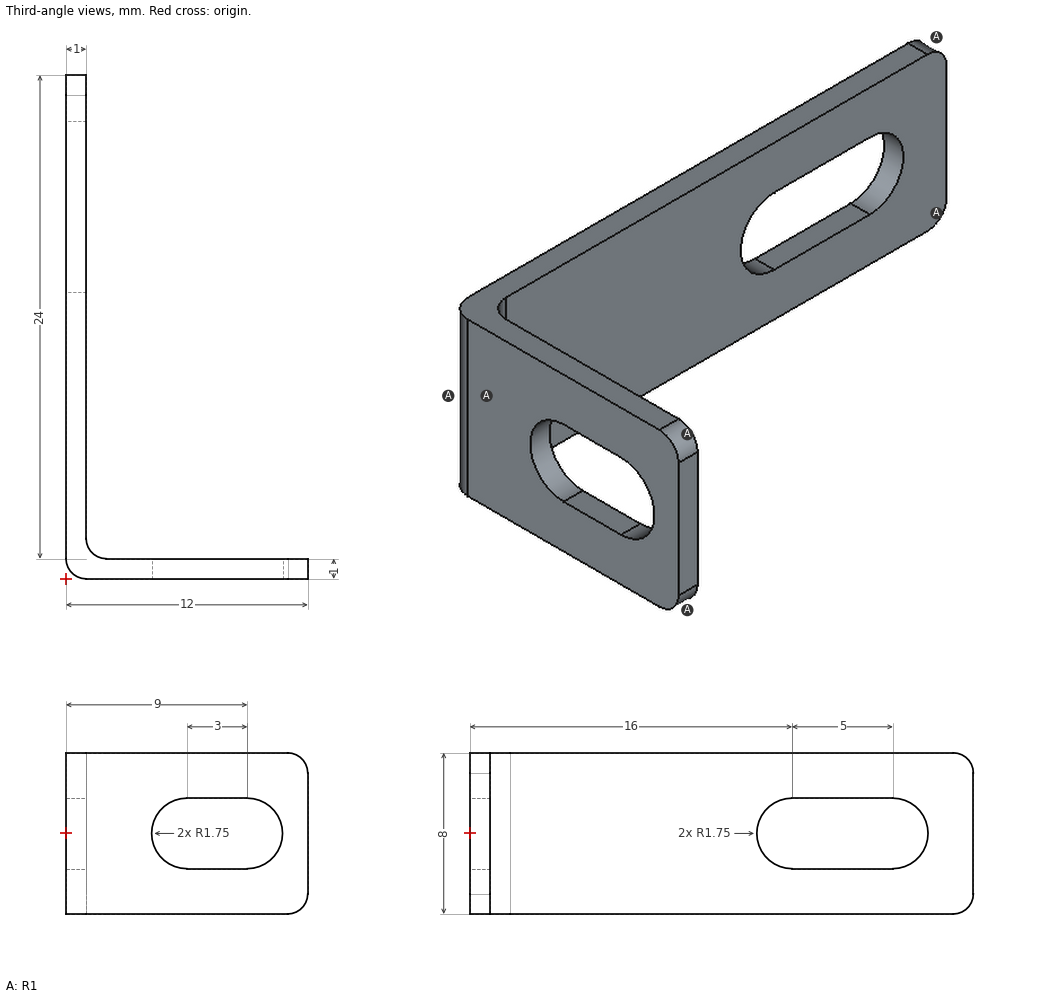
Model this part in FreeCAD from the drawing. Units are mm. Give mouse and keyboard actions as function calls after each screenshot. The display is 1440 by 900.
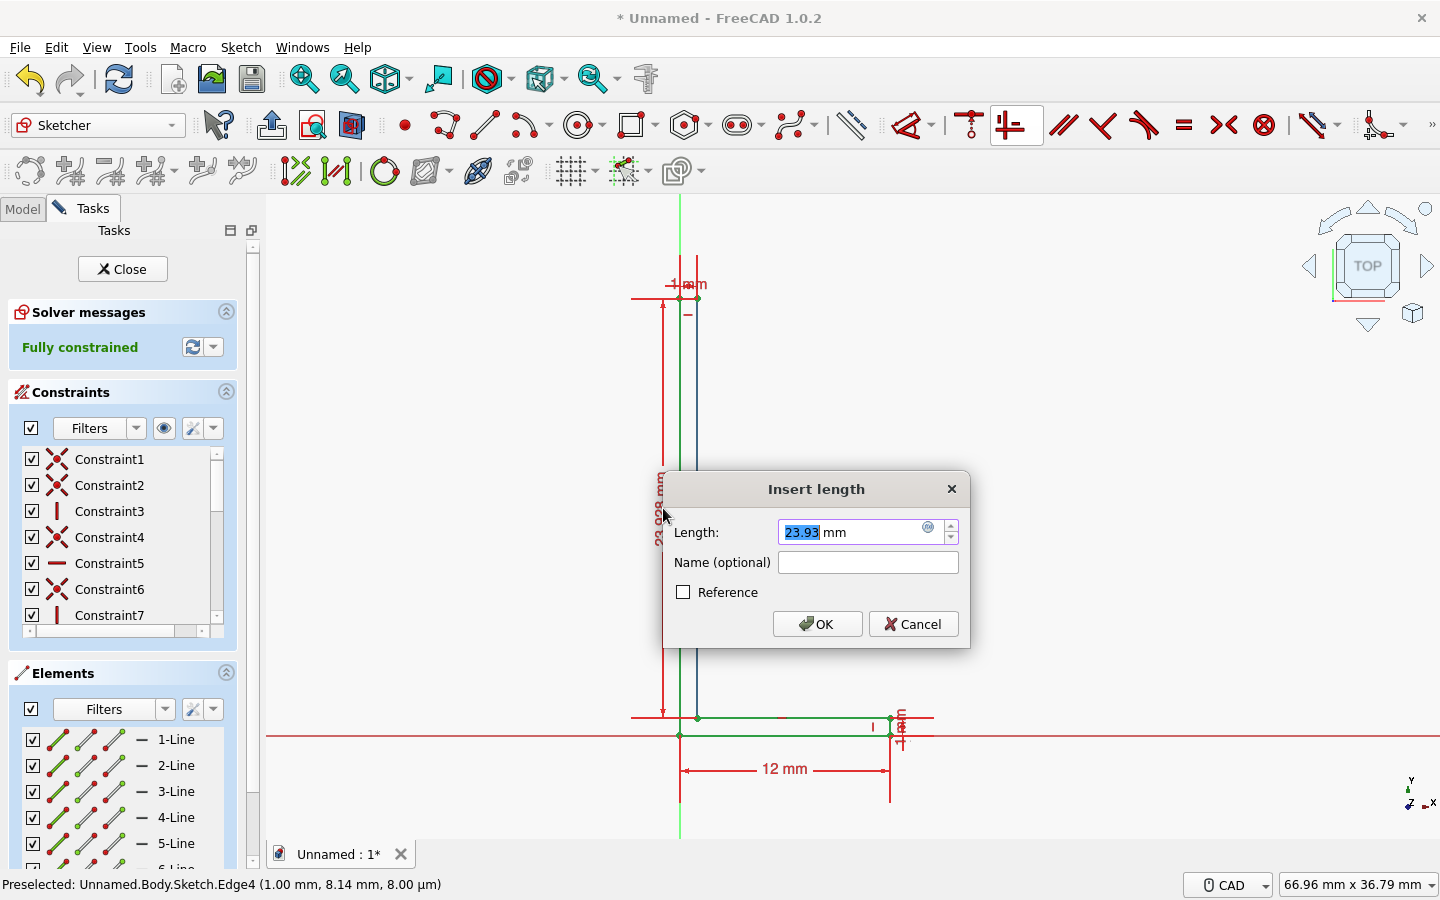
text(24)
key(Return)
key(Escape)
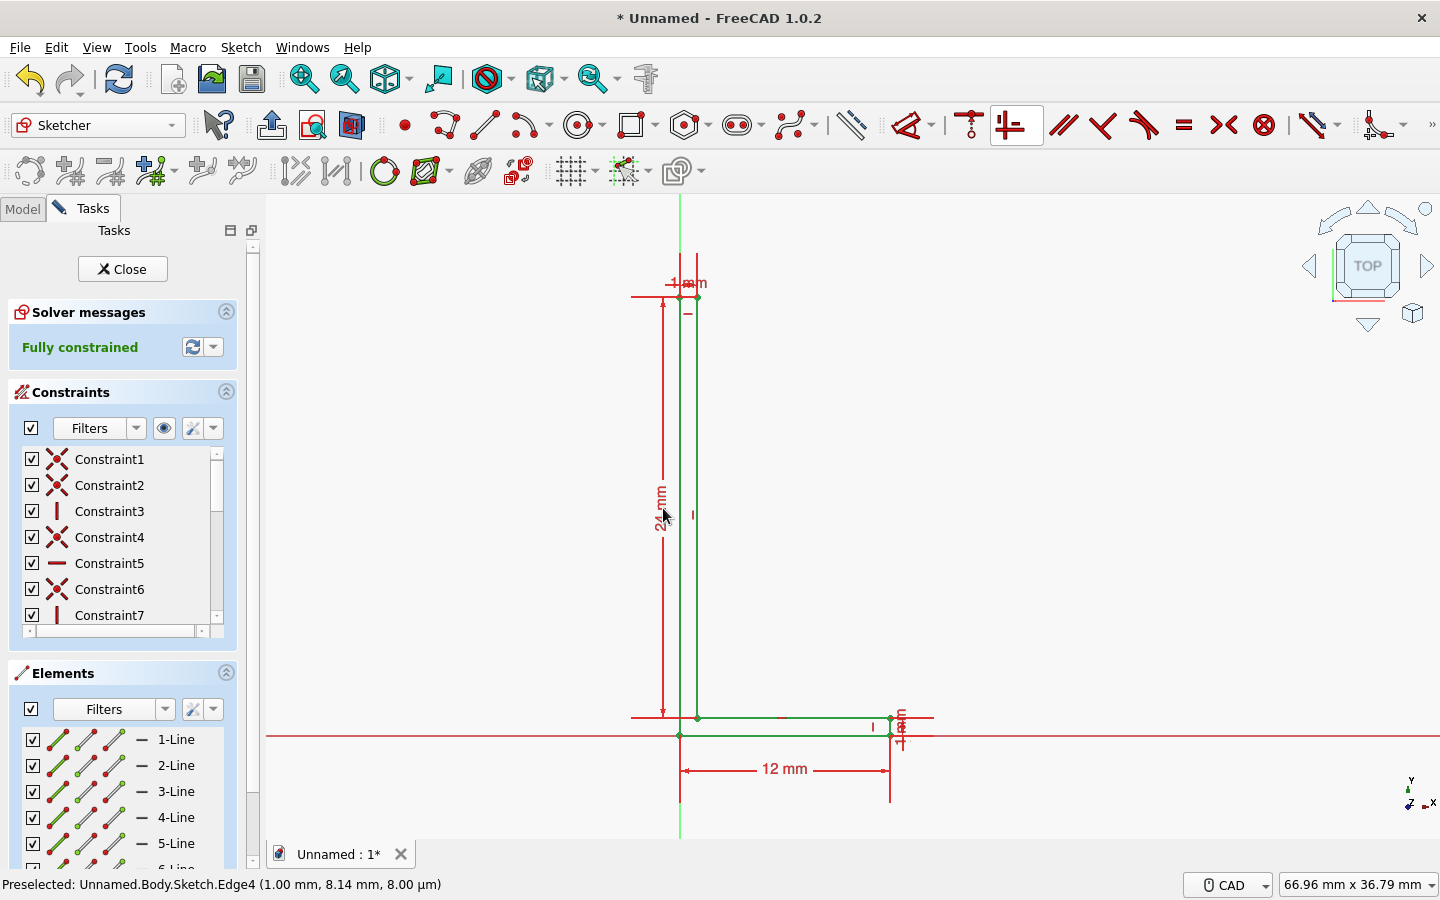
click(123, 269)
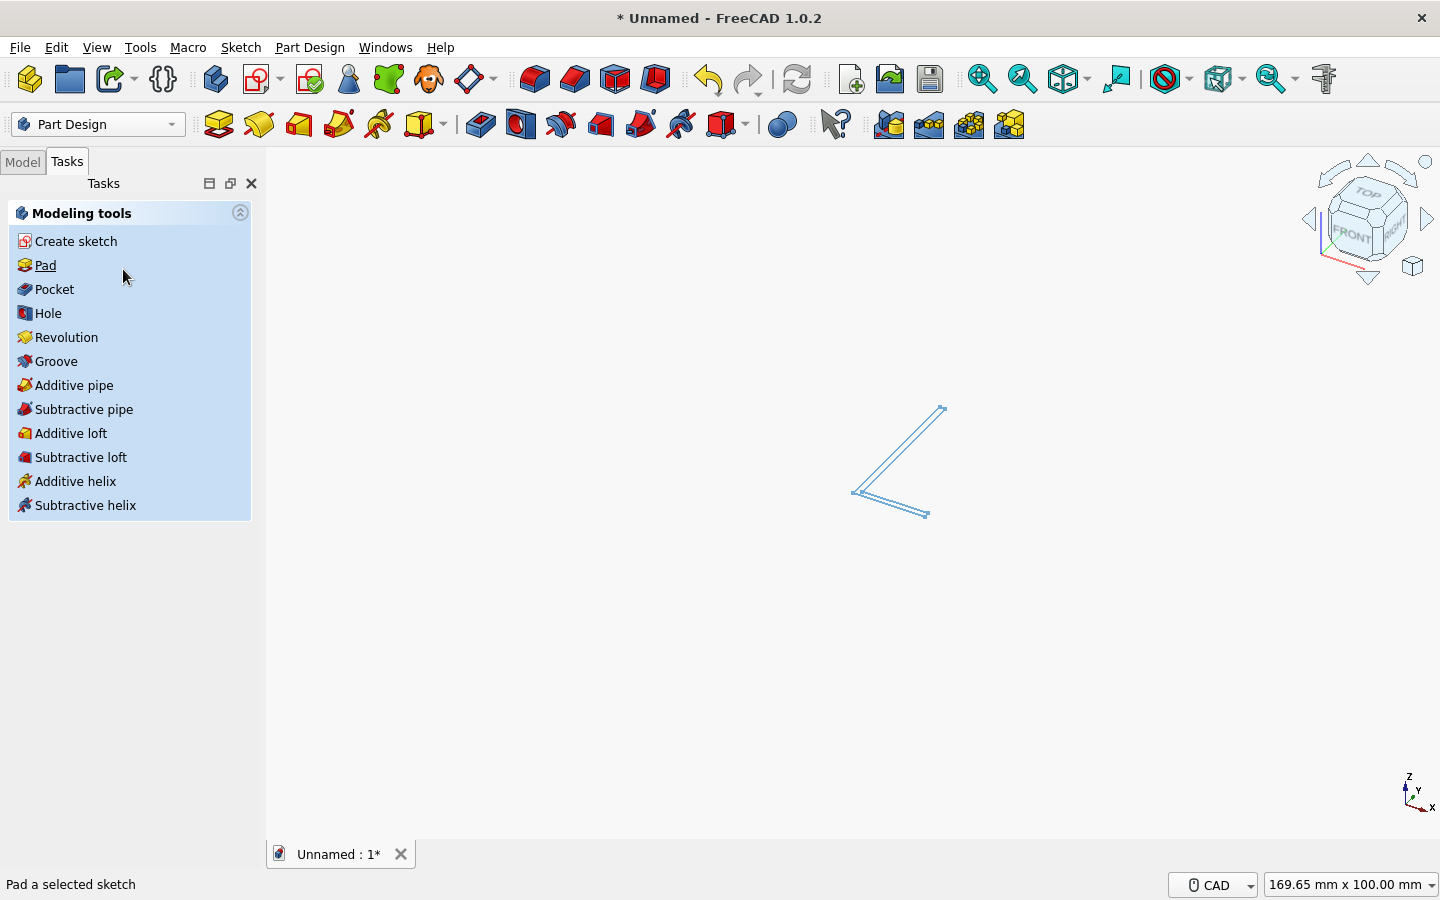
click(220, 124)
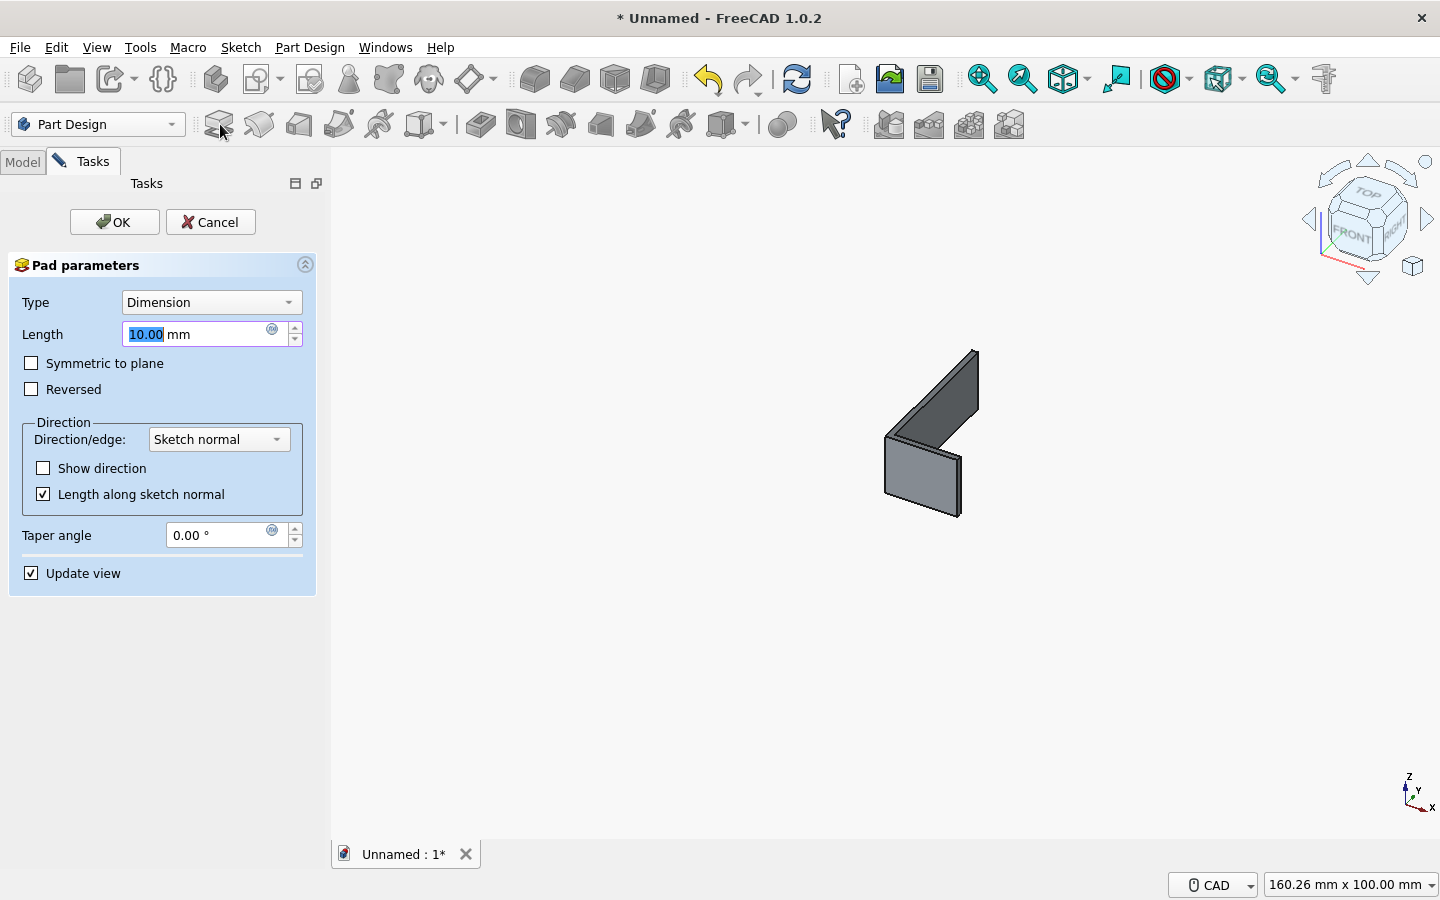
text(8)
key(Tab)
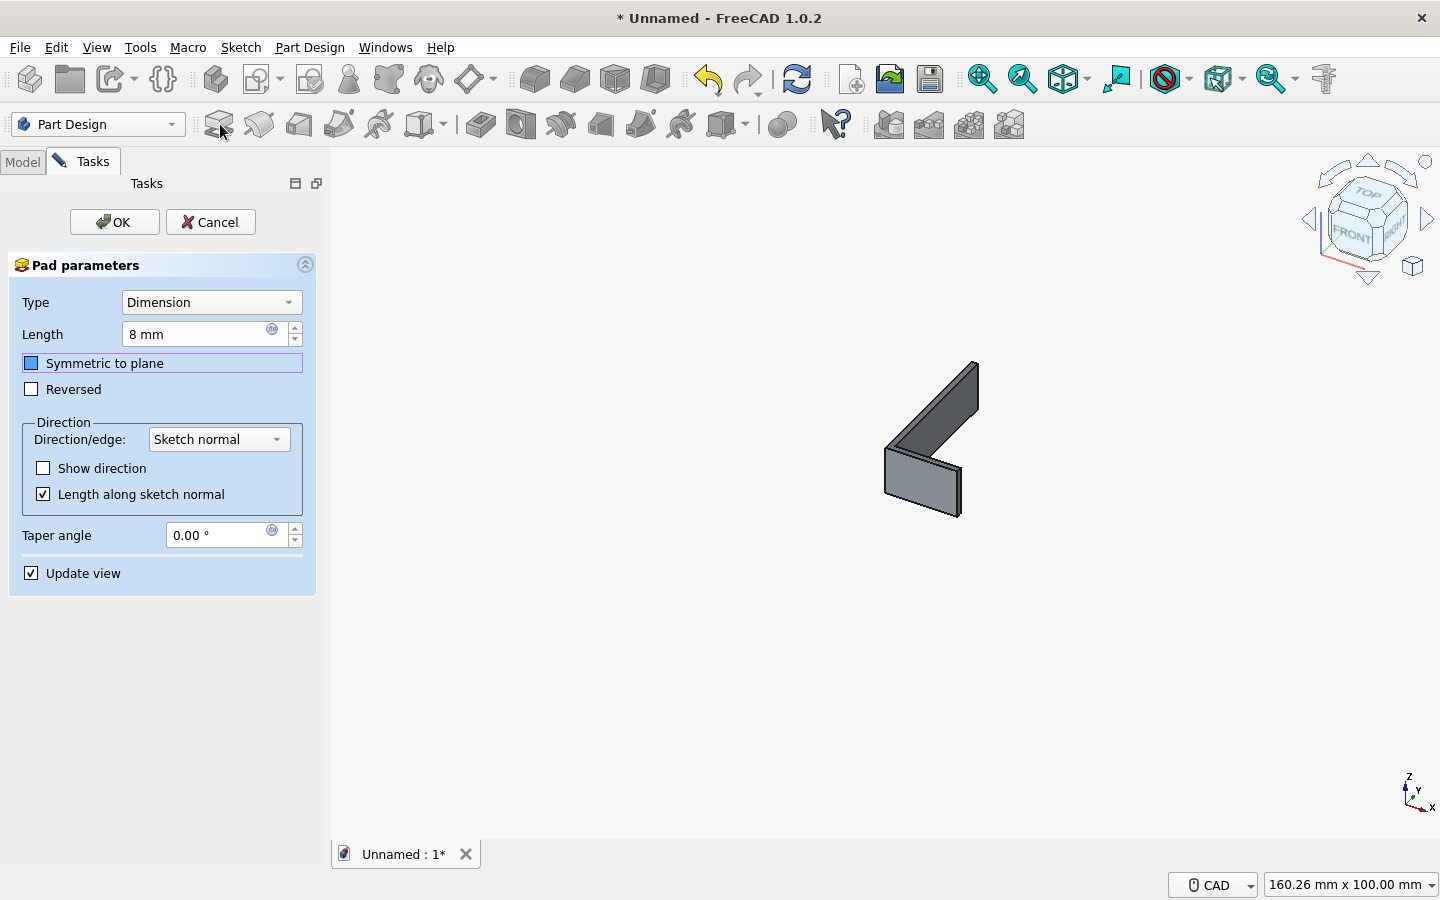
click(30, 363)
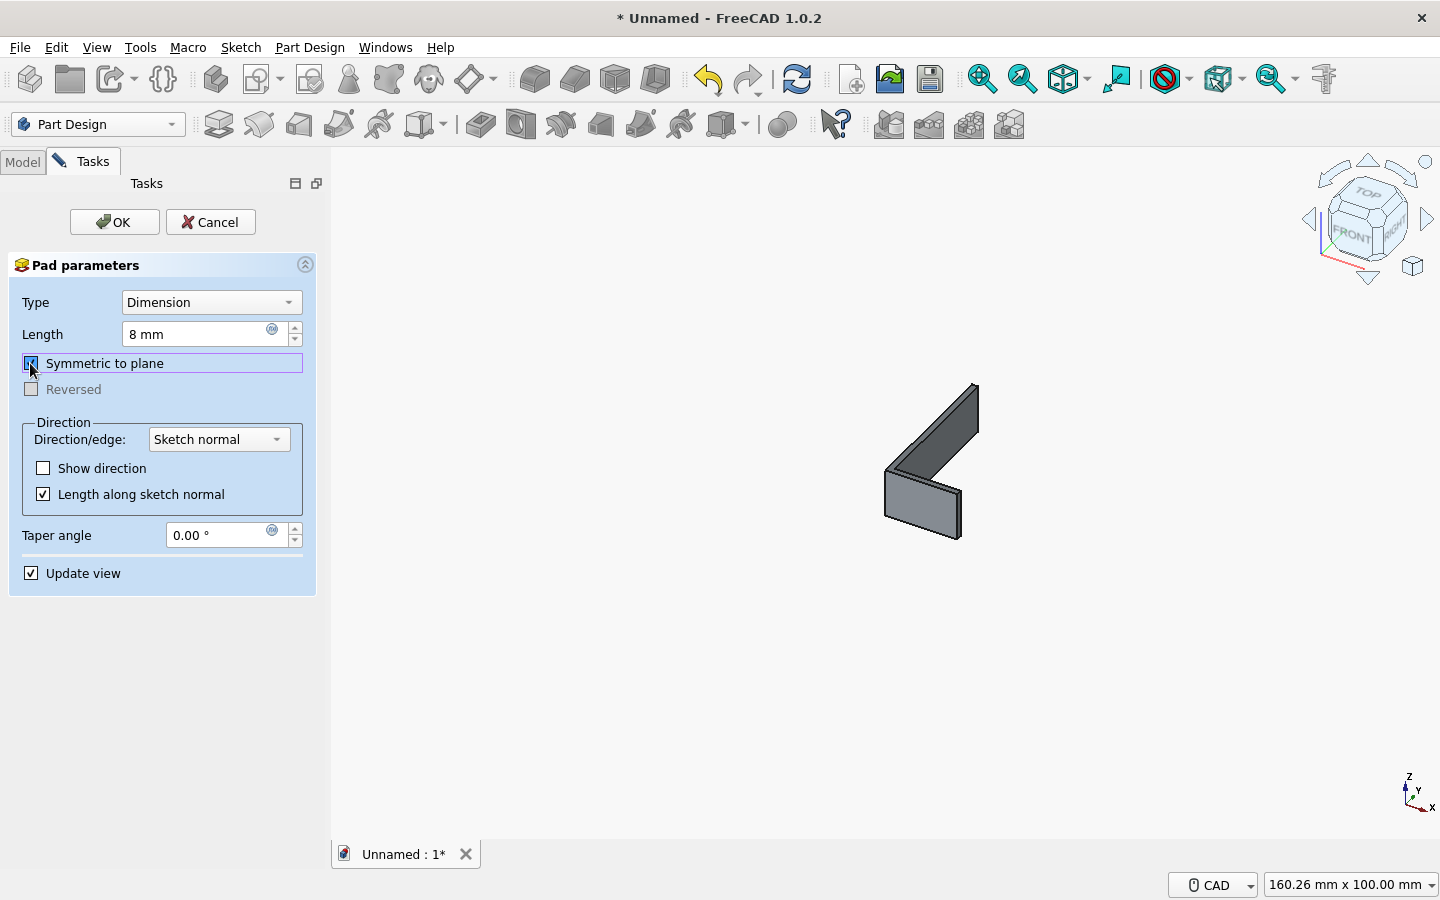
click(115, 222)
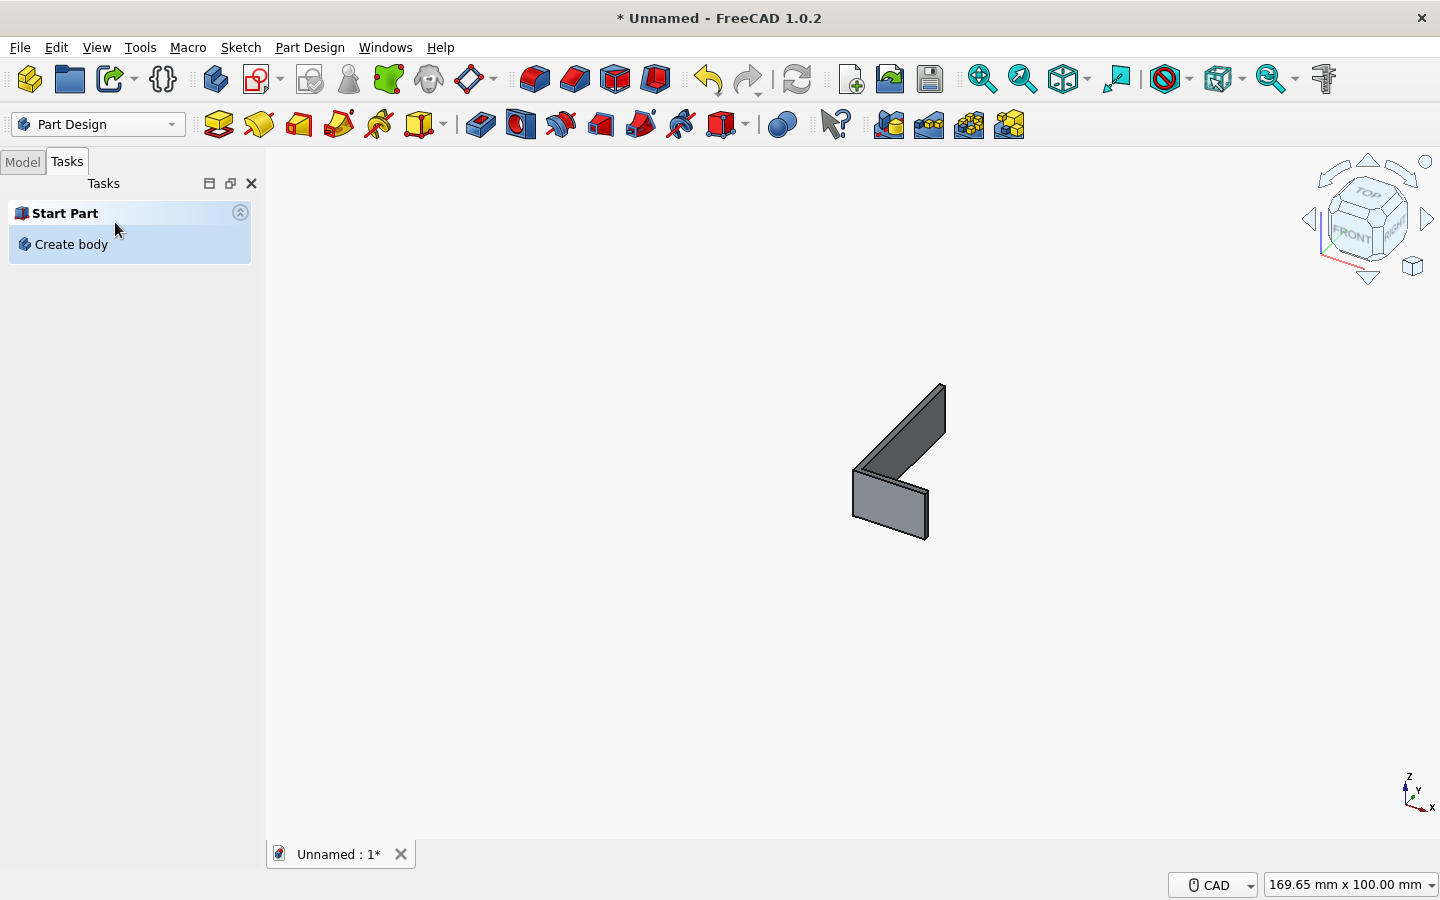
key(v)
key(f)